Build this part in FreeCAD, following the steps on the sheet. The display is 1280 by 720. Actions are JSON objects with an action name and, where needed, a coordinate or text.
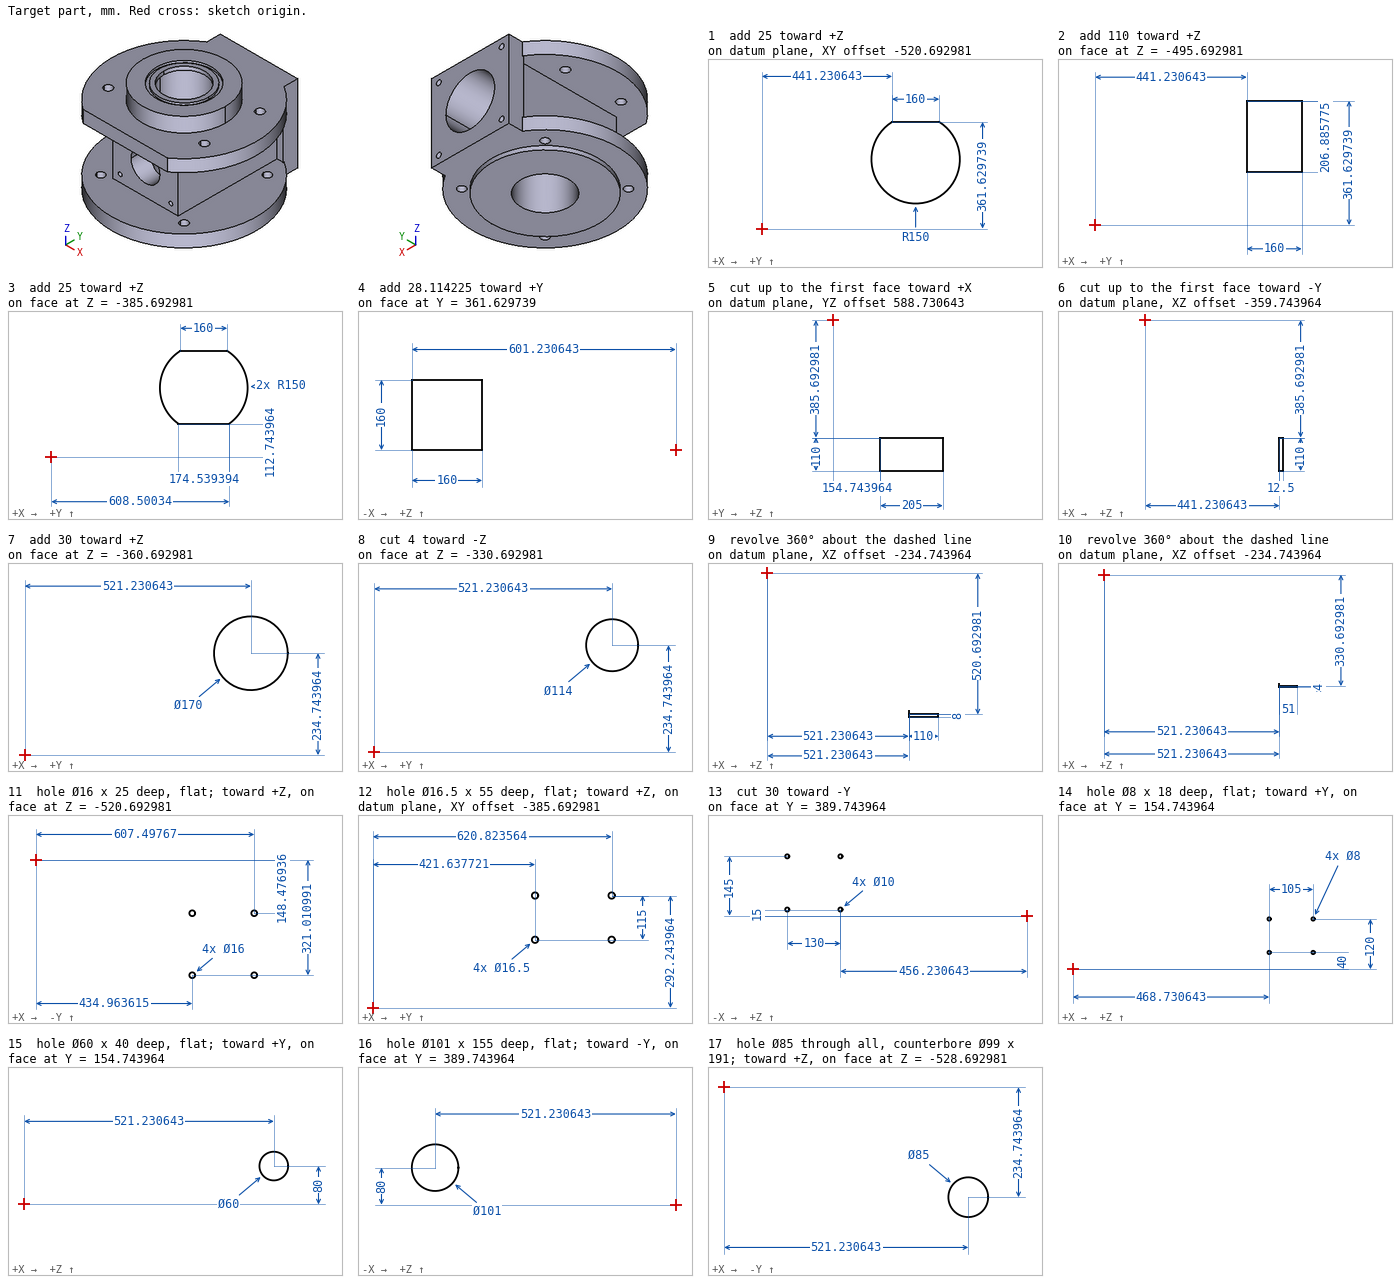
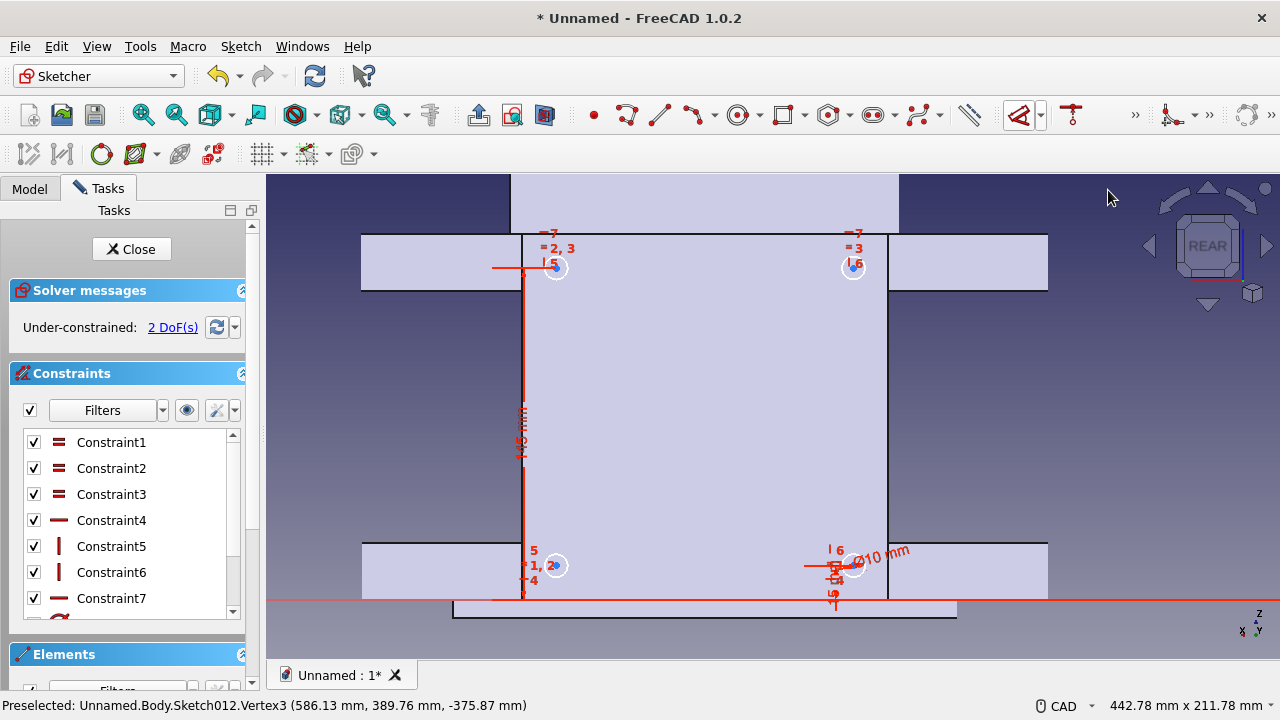
{"action": "left_click", "coordinate": [854, 566]}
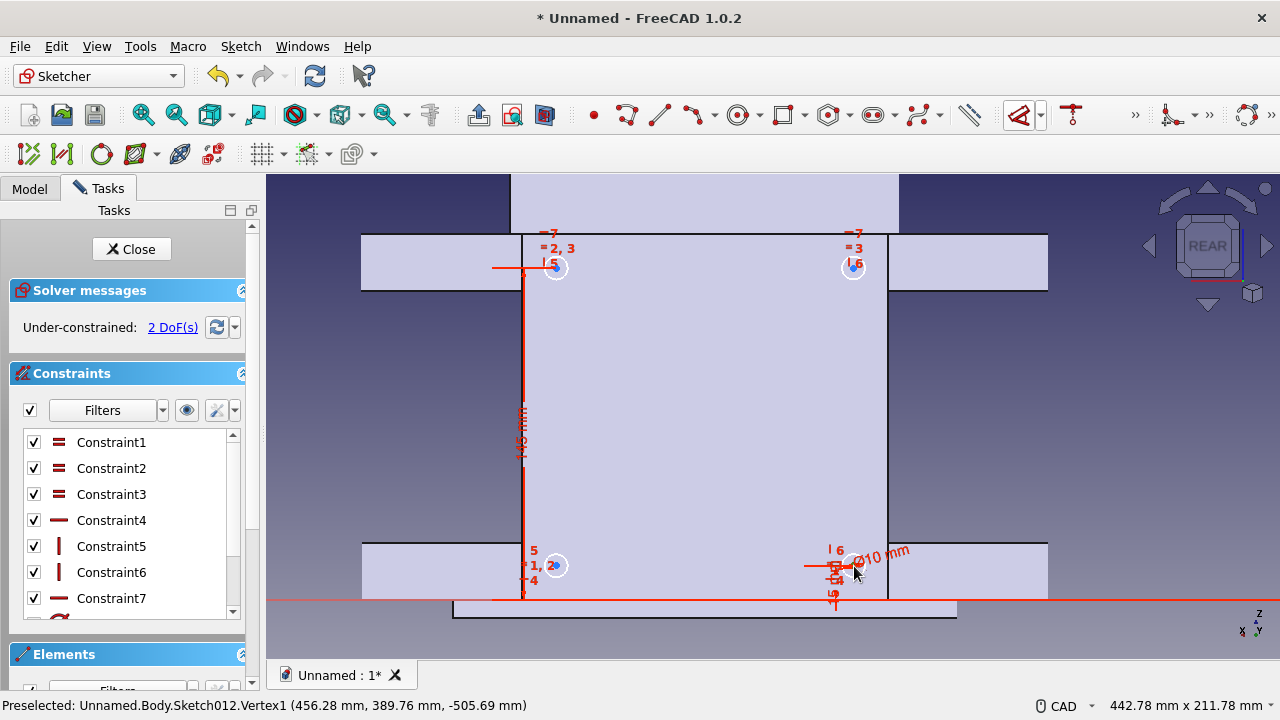
{"action": "left_click", "coordinate": [556, 566]}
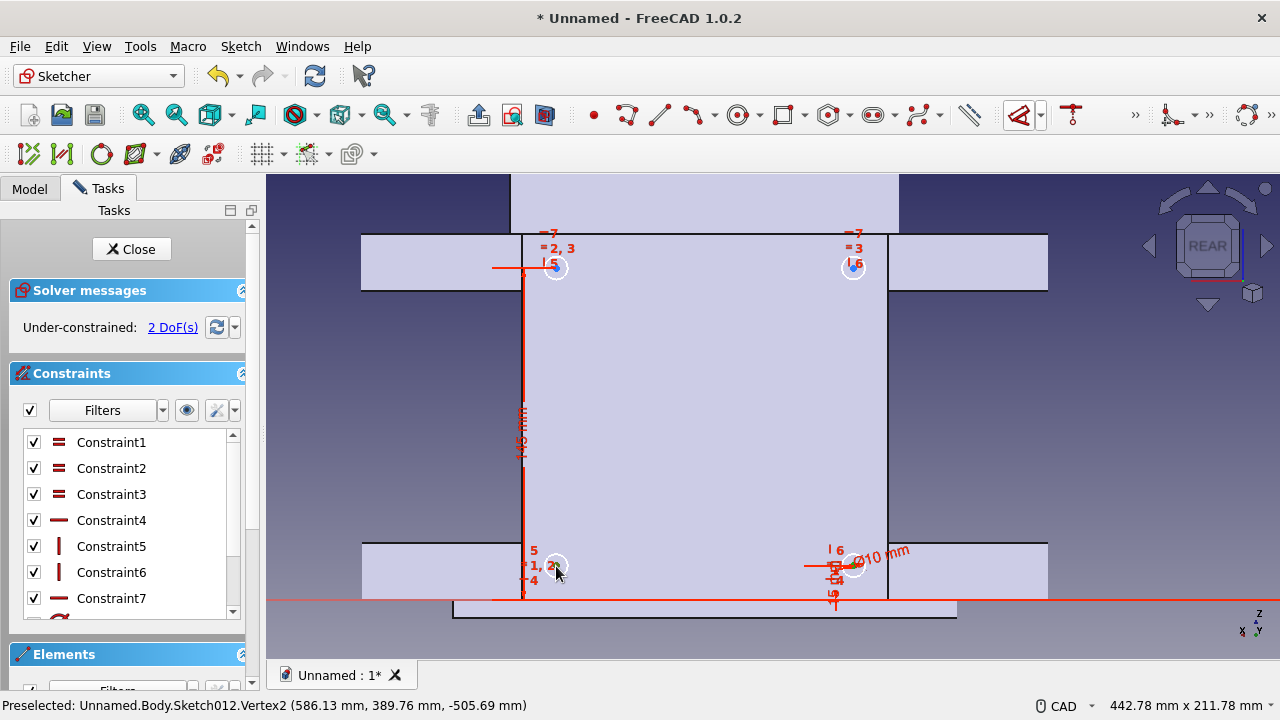
{"action": "left_click", "coordinate": [1040, 116]}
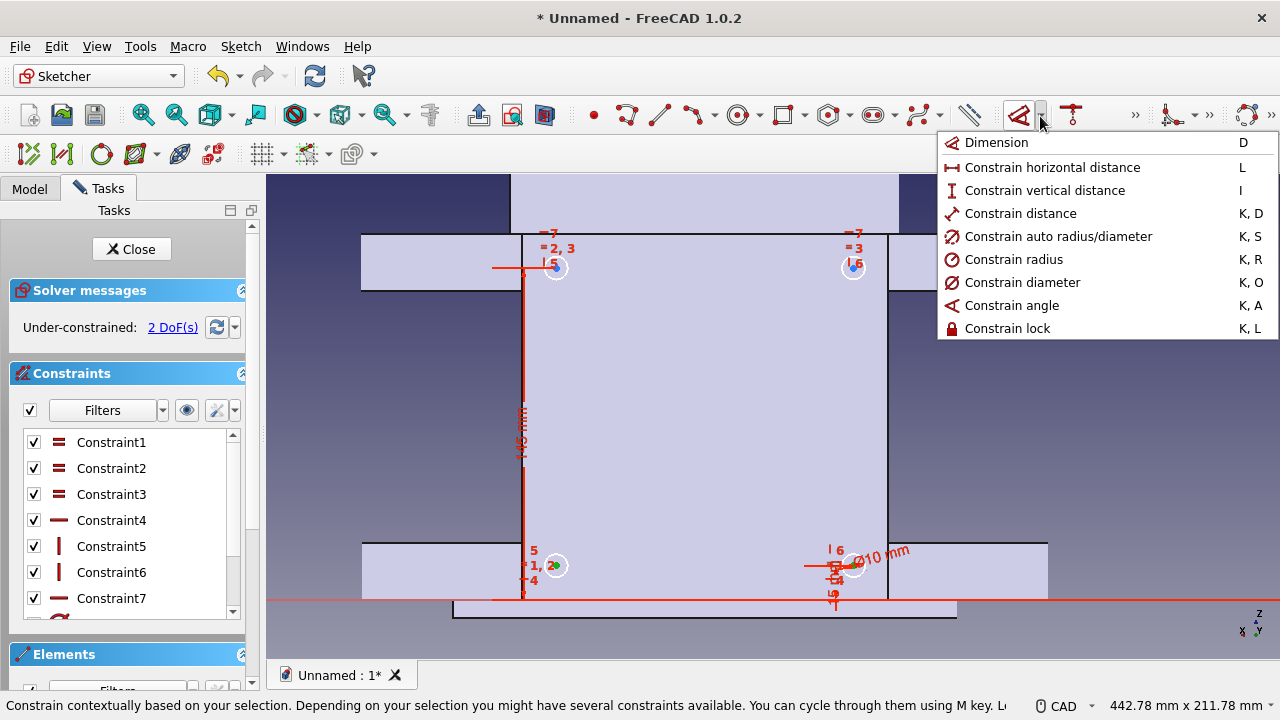
{"action": "left_click", "coordinate": [1108, 168]}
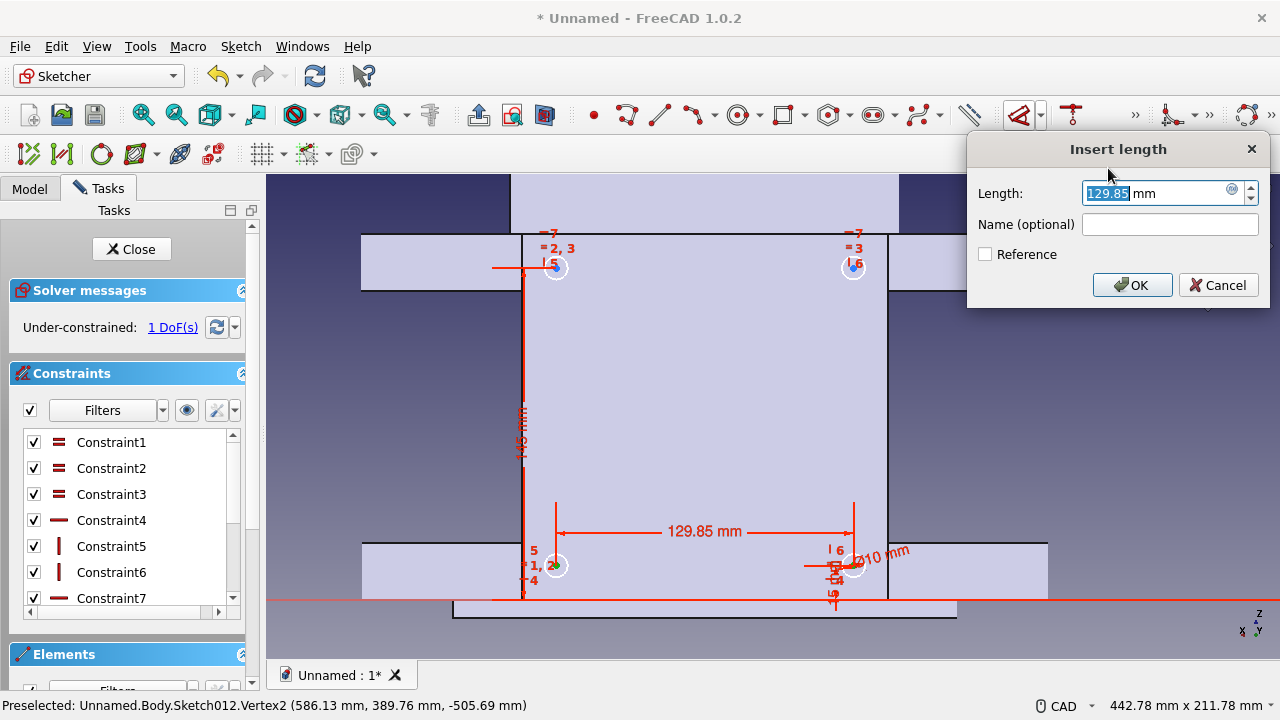
{"action": "type", "text": "130"}
{"action": "key", "text": "Return"}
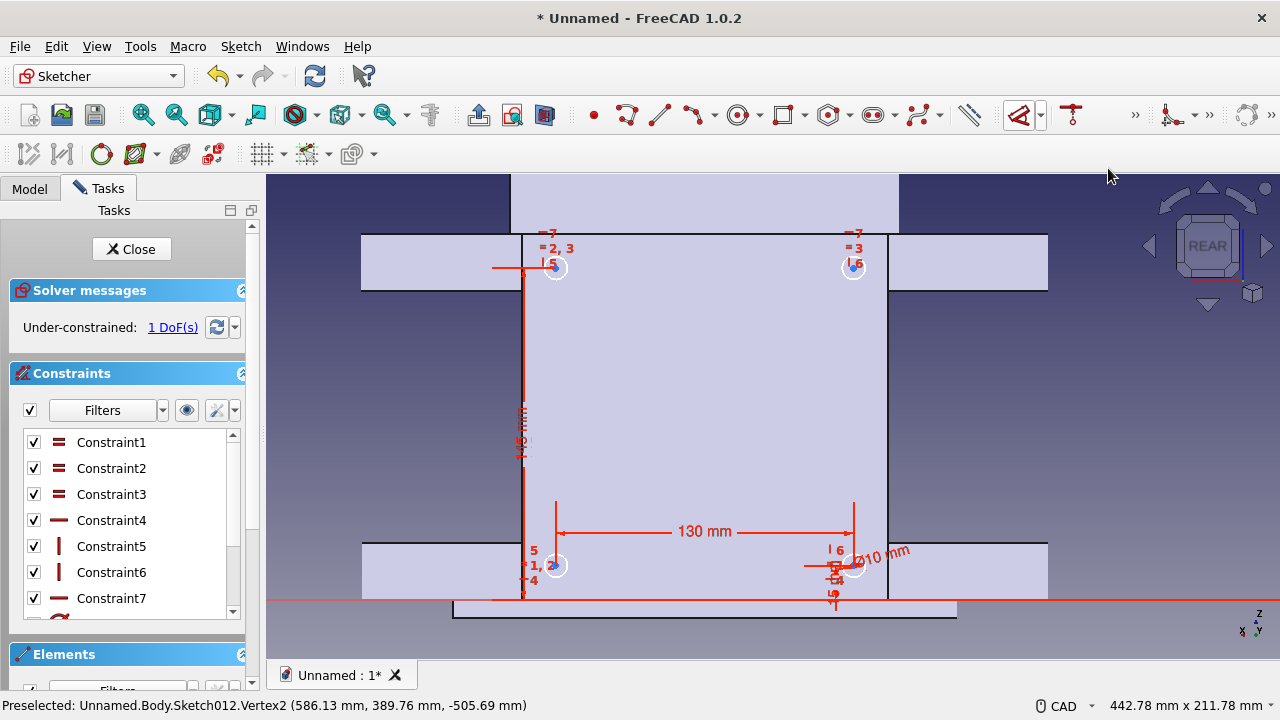
{"action": "left_click", "coordinate": [854, 566]}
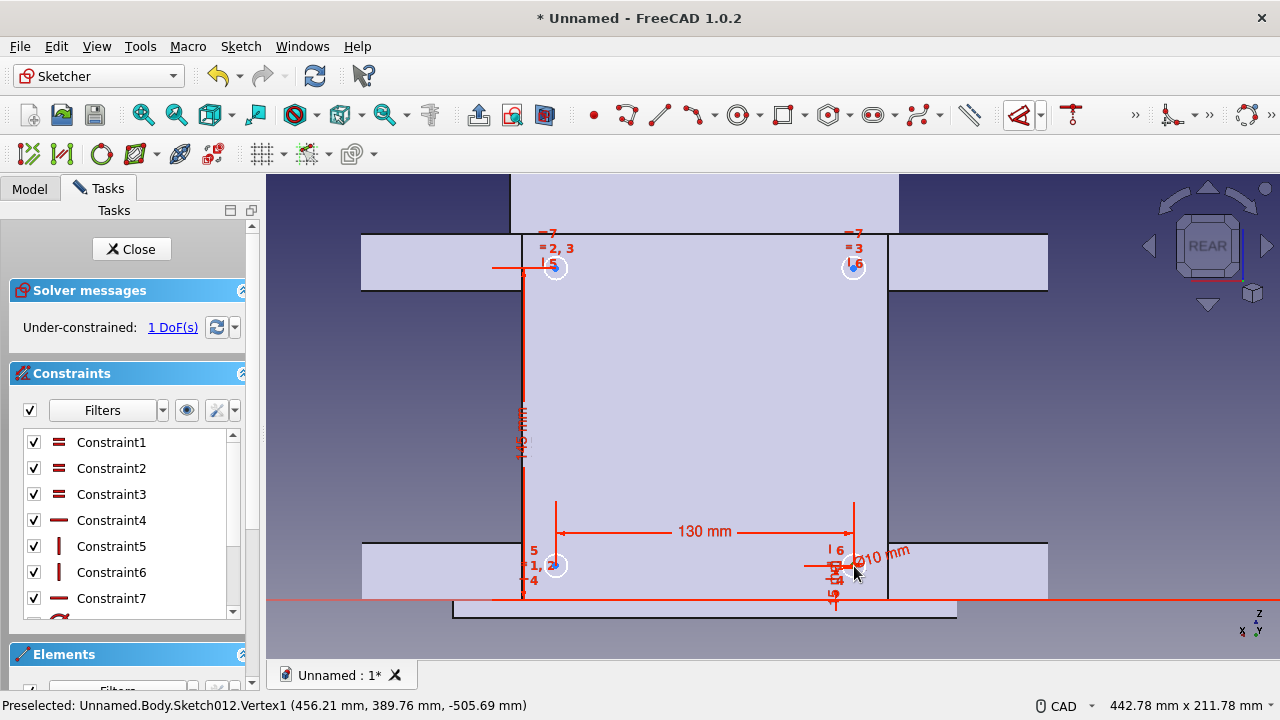
{"action": "key", "text": "l"}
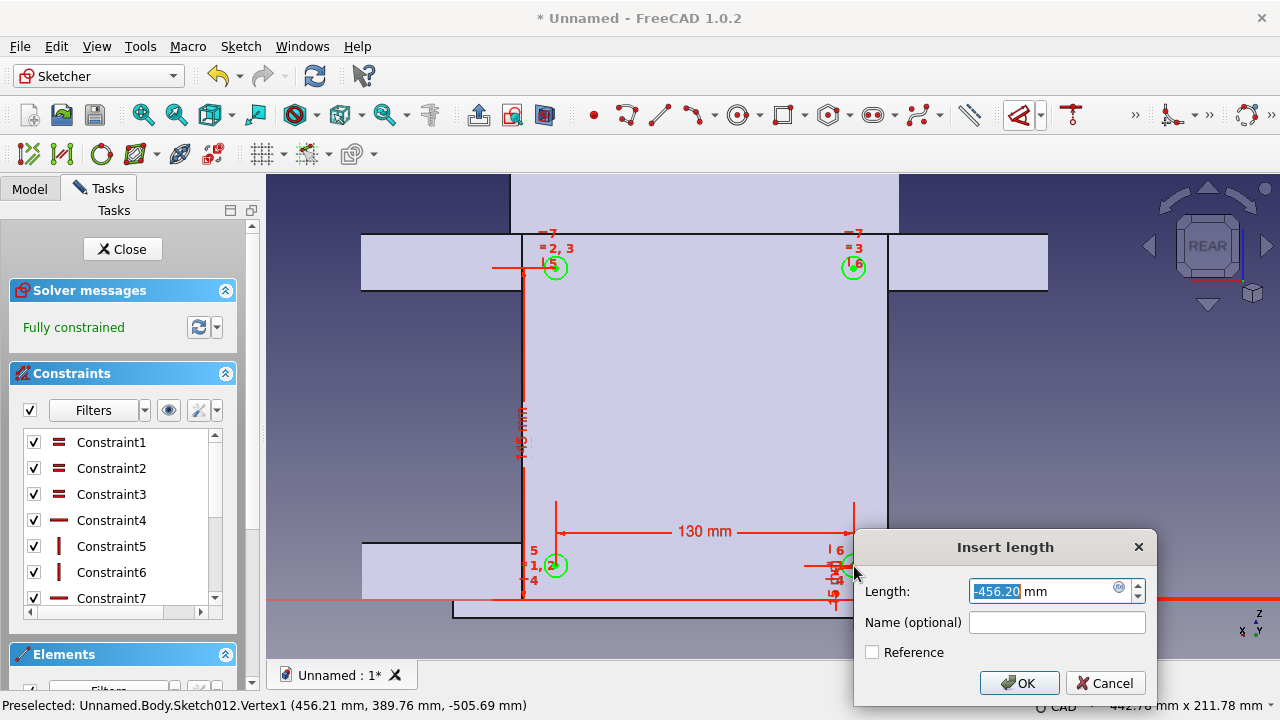
{"action": "type", "text": "-456.230643"}
{"action": "key", "text": "Return"}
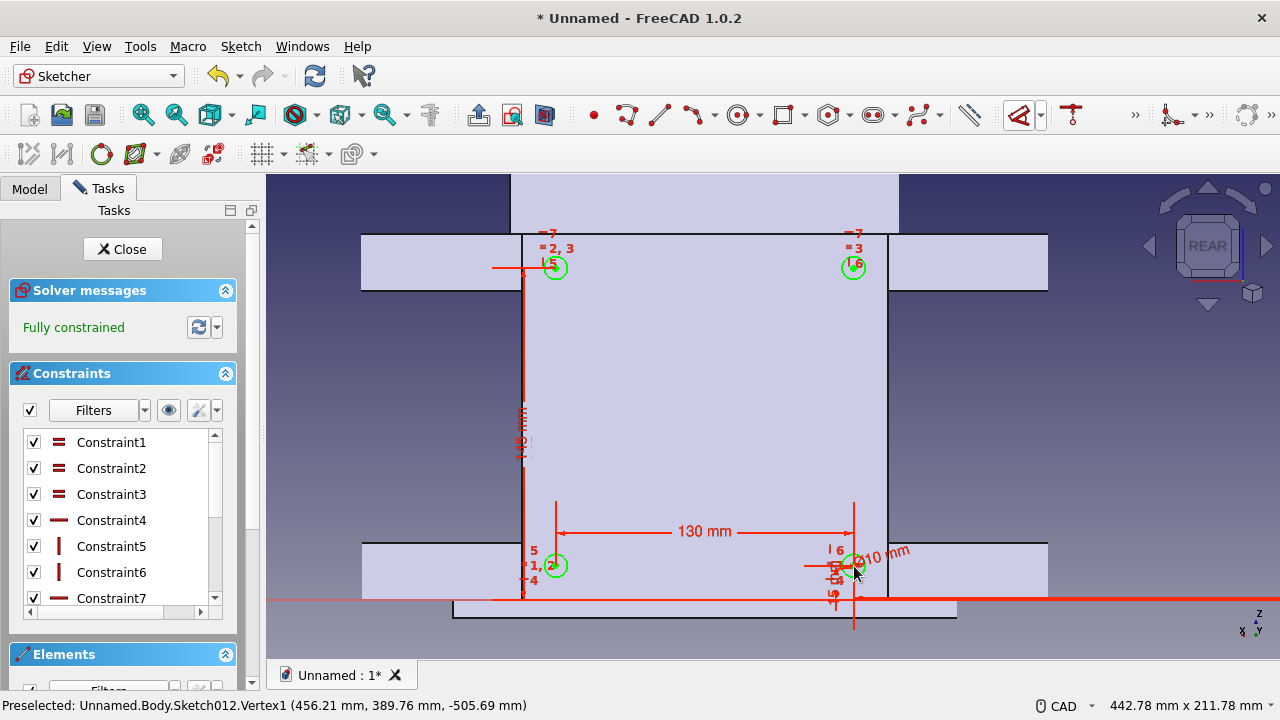
{"action": "left_click", "coordinate": [123, 249]}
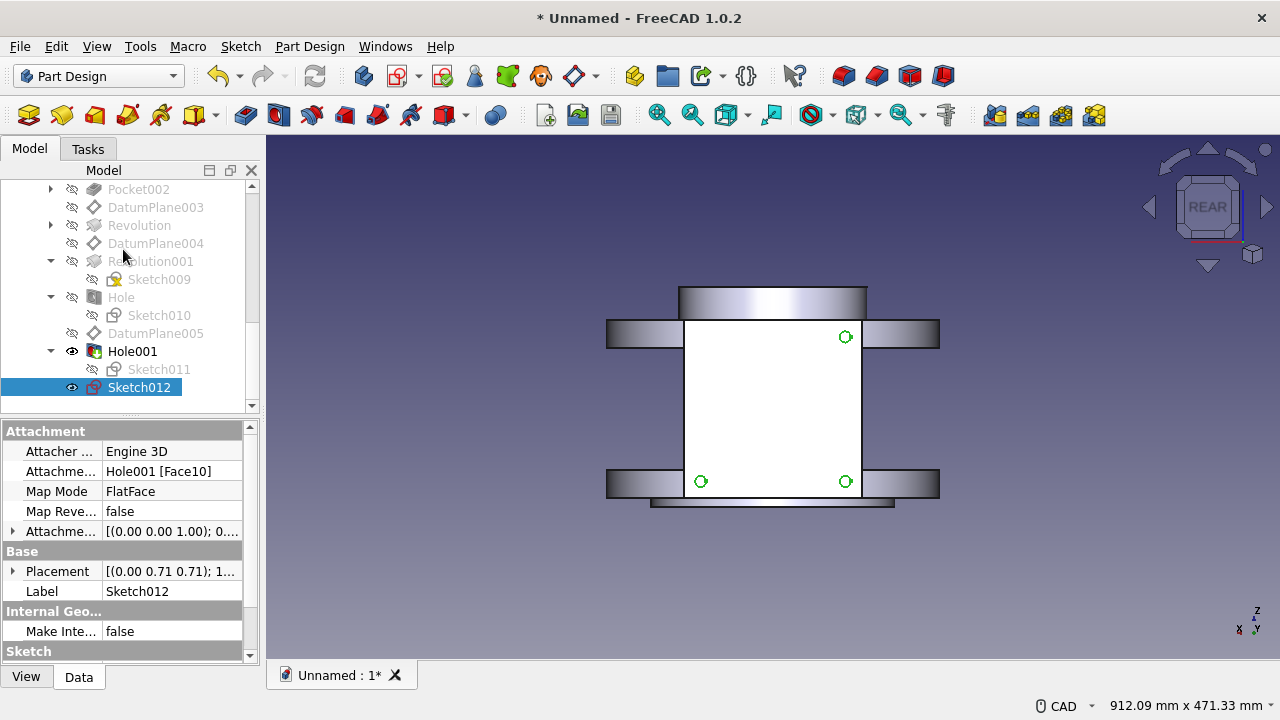
{"action": "left_click", "coordinate": [246, 116]}